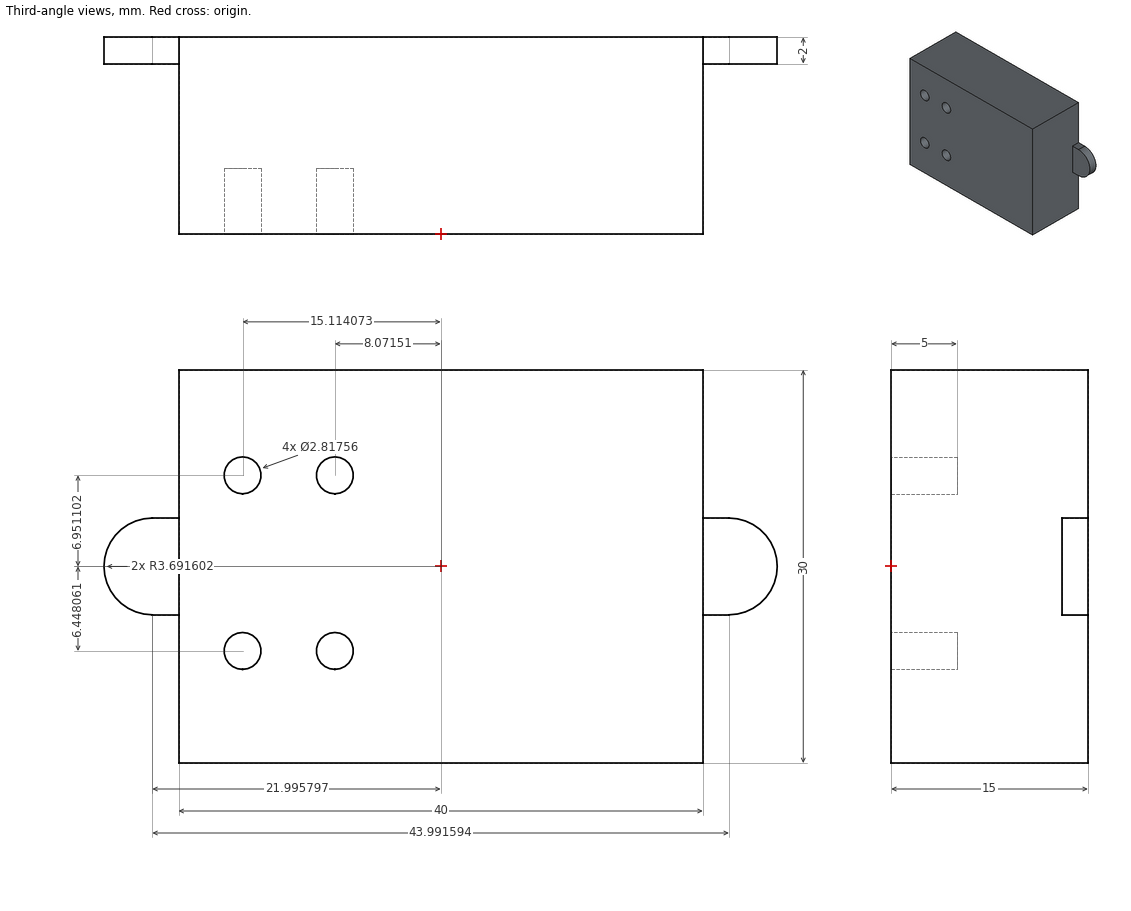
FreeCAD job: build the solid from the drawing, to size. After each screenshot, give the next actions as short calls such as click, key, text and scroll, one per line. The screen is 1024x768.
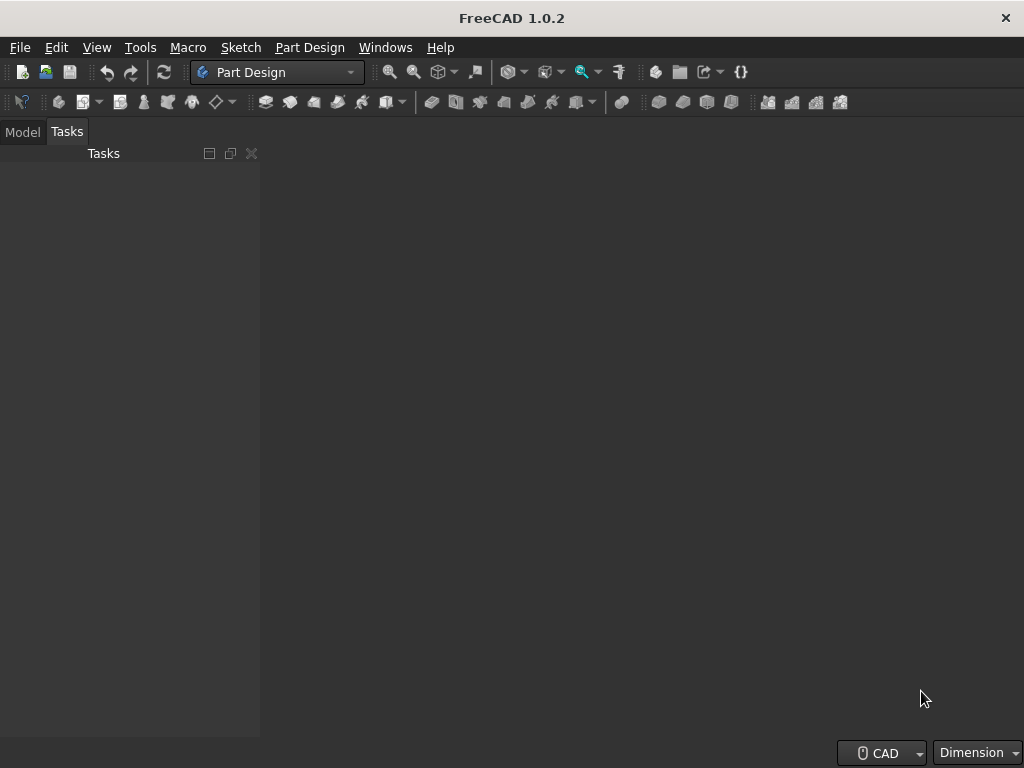
click(524, 72)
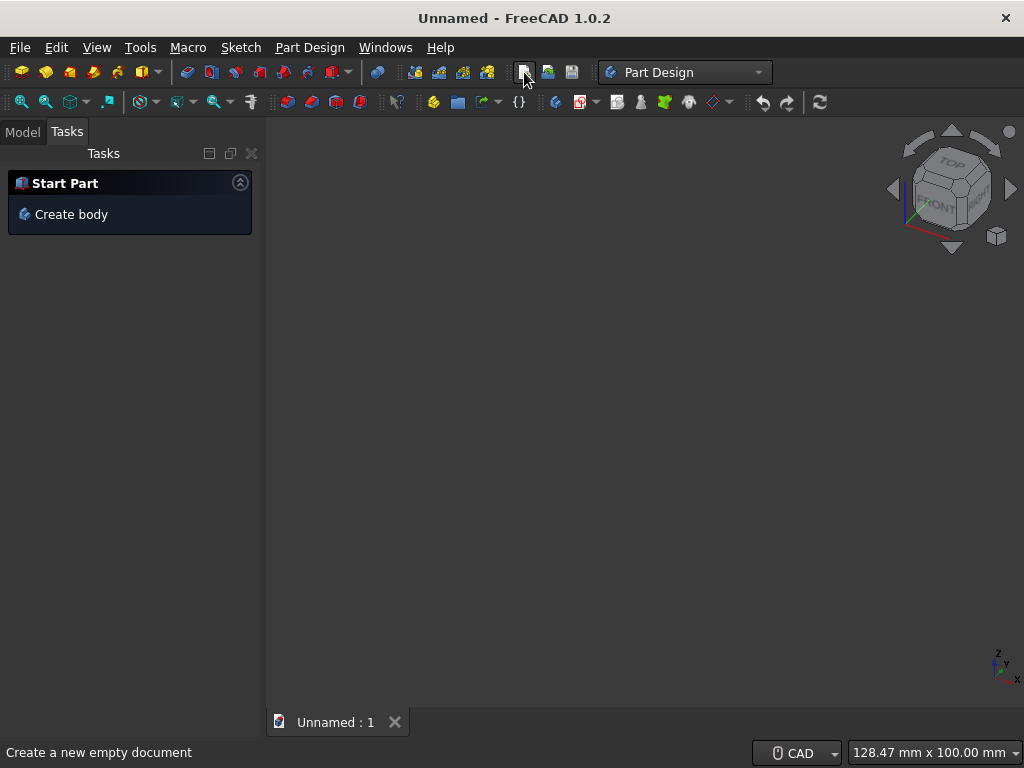
click(580, 102)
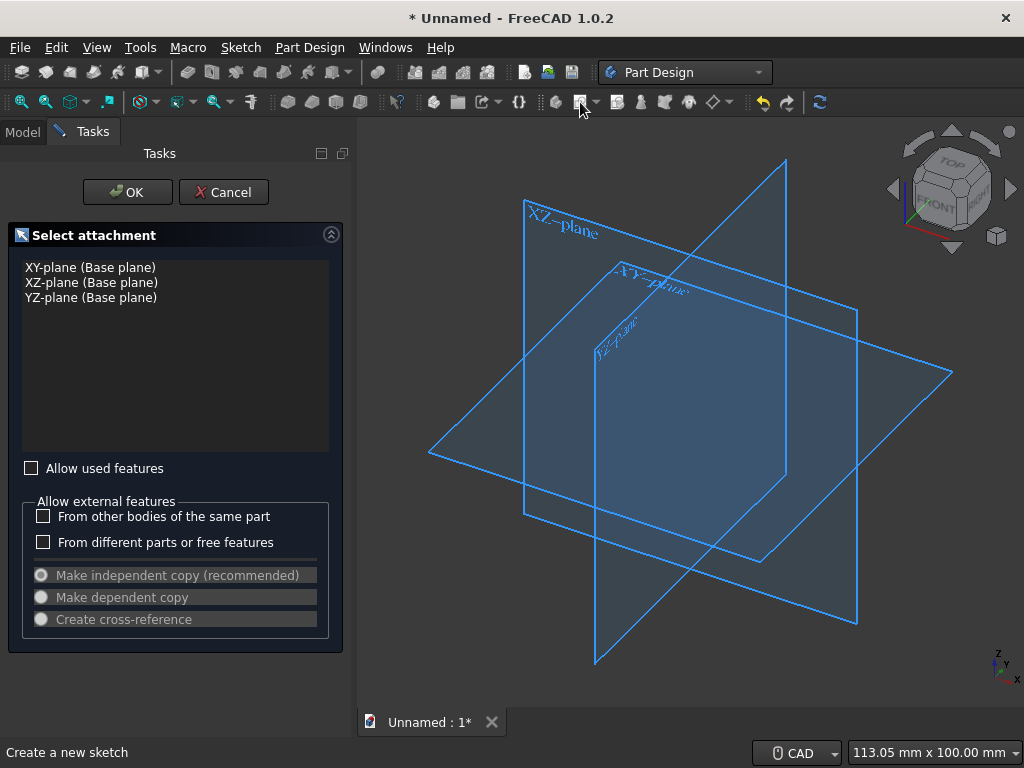
click(82, 282)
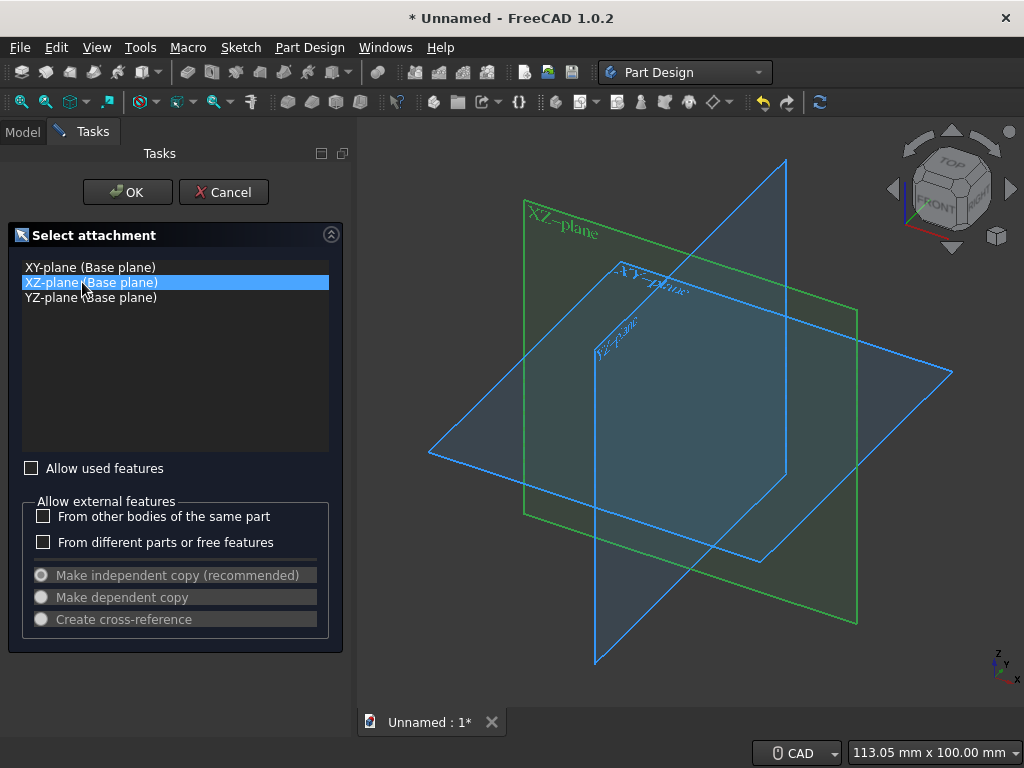
click(128, 192)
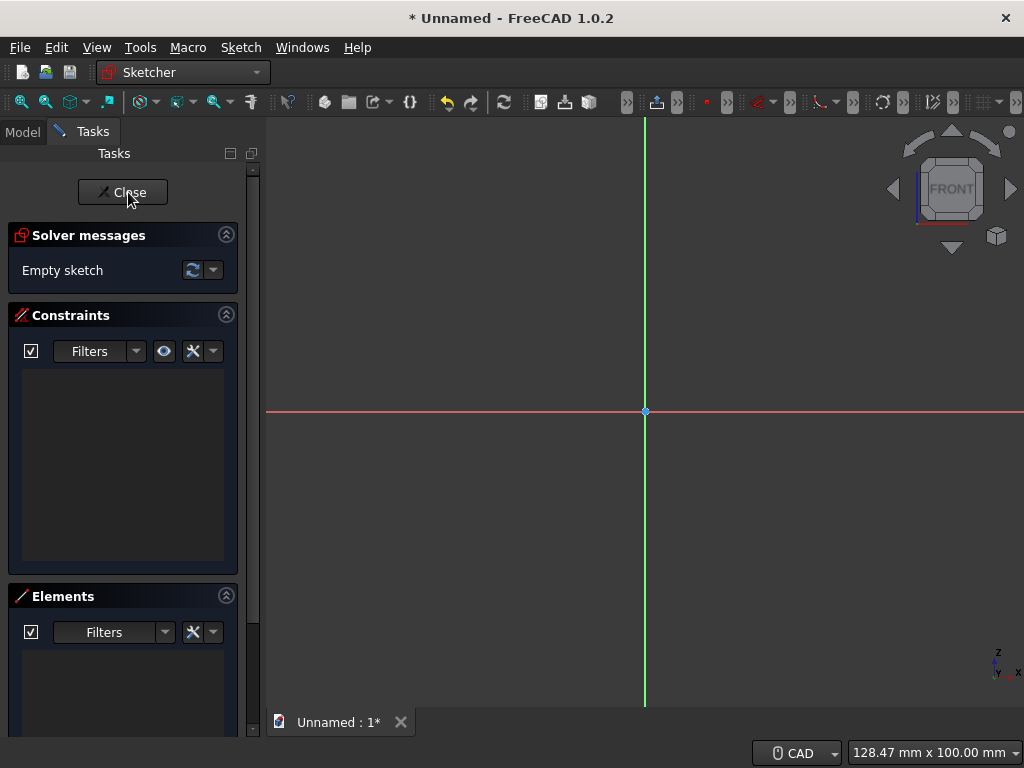
scroll(728, 412, up, 3)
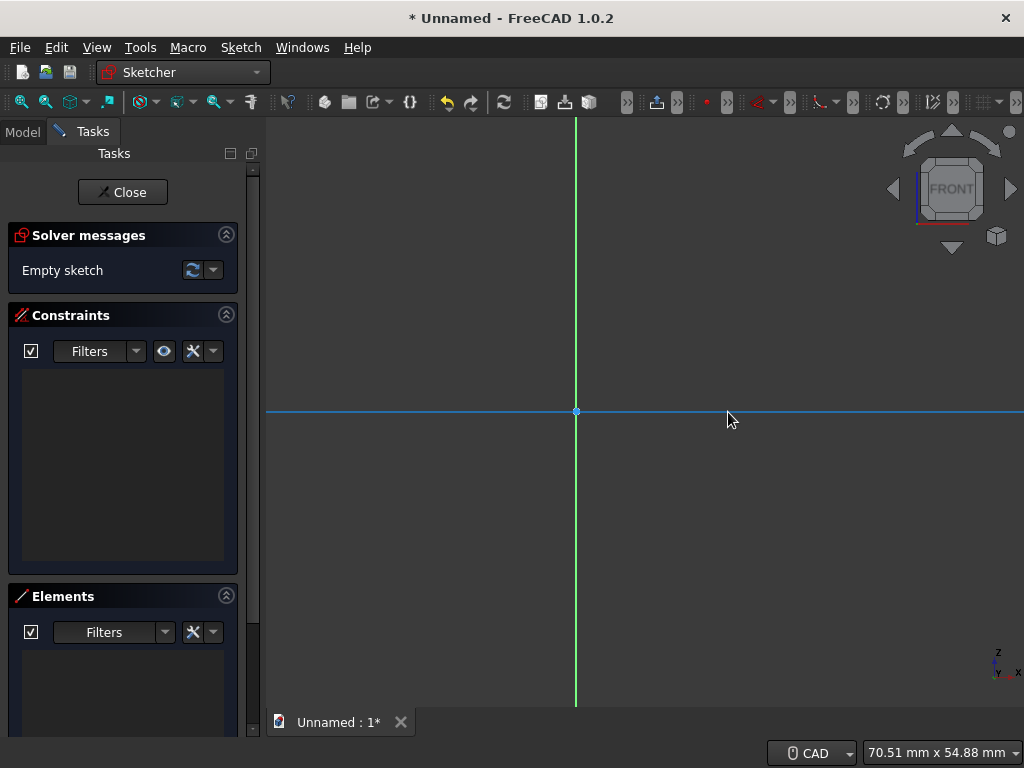
key(g)
key(v)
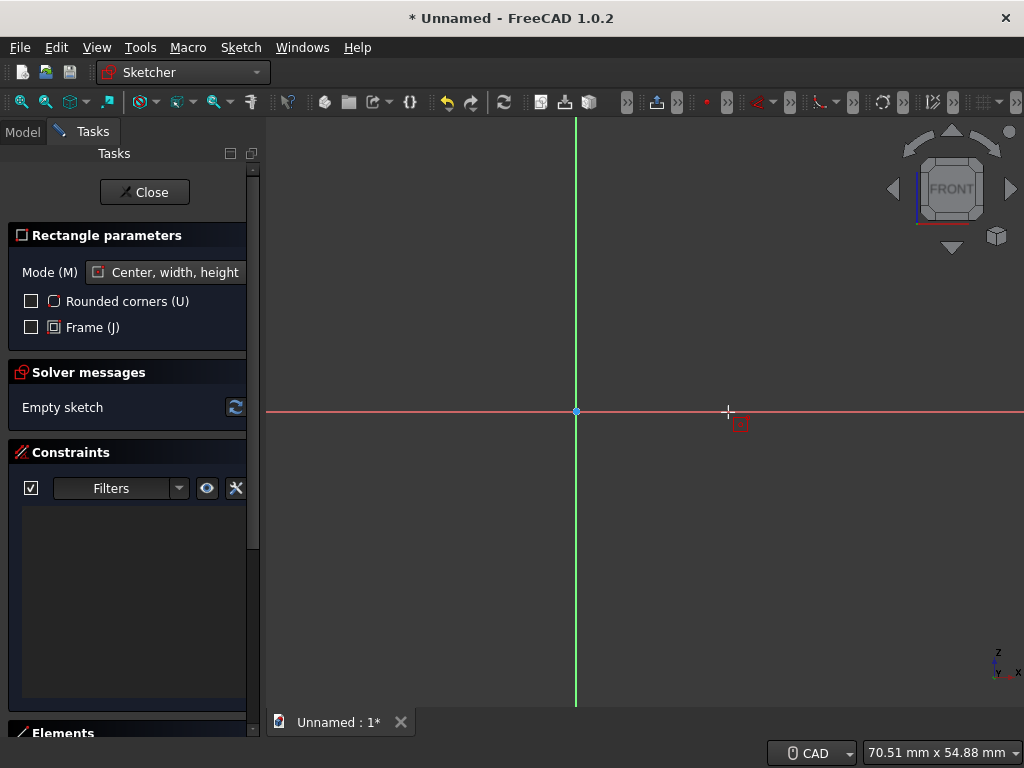
click(576, 412)
click(791, 250)
key(Escape)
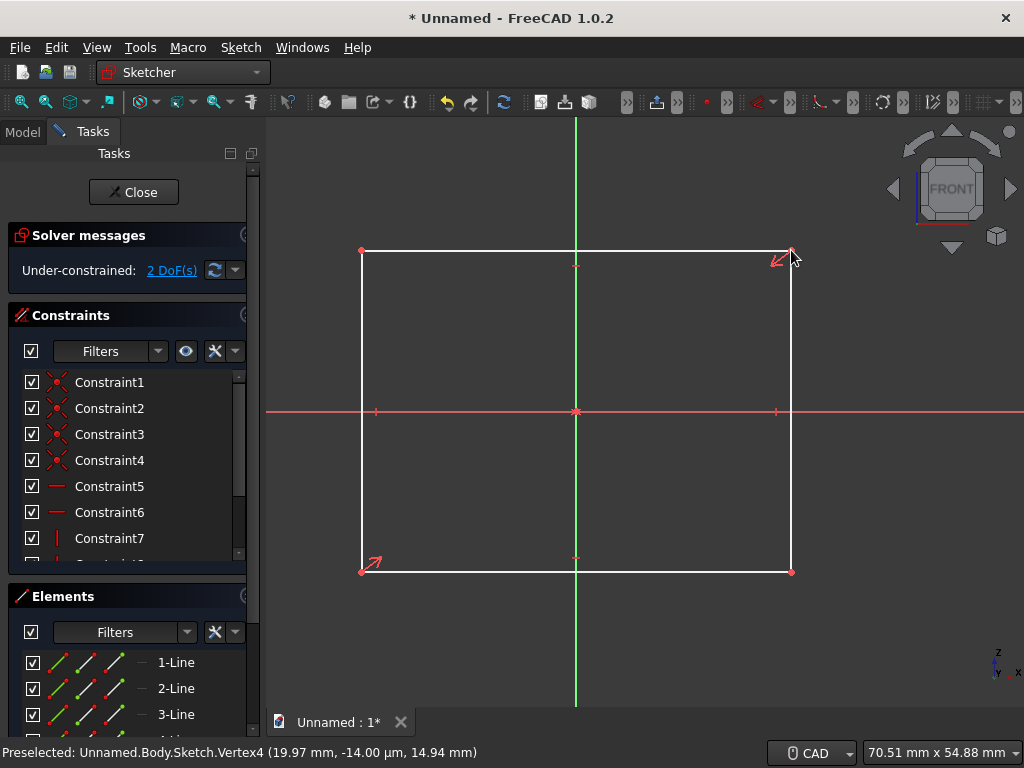
key(d)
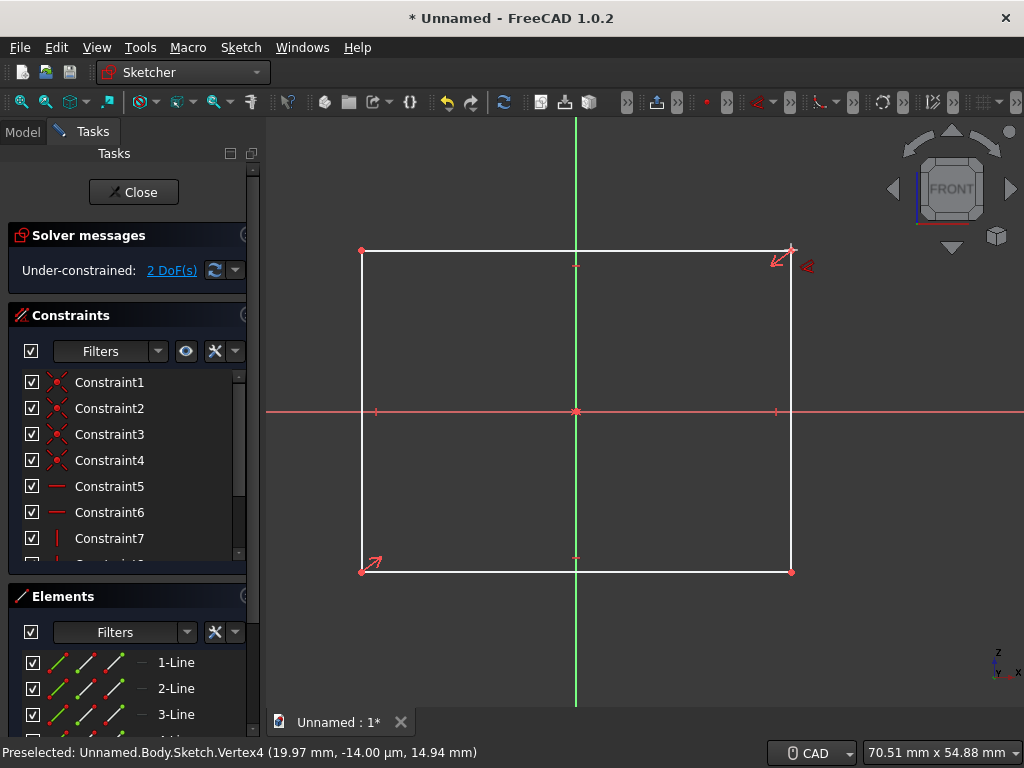
click(490, 572)
click(477, 606)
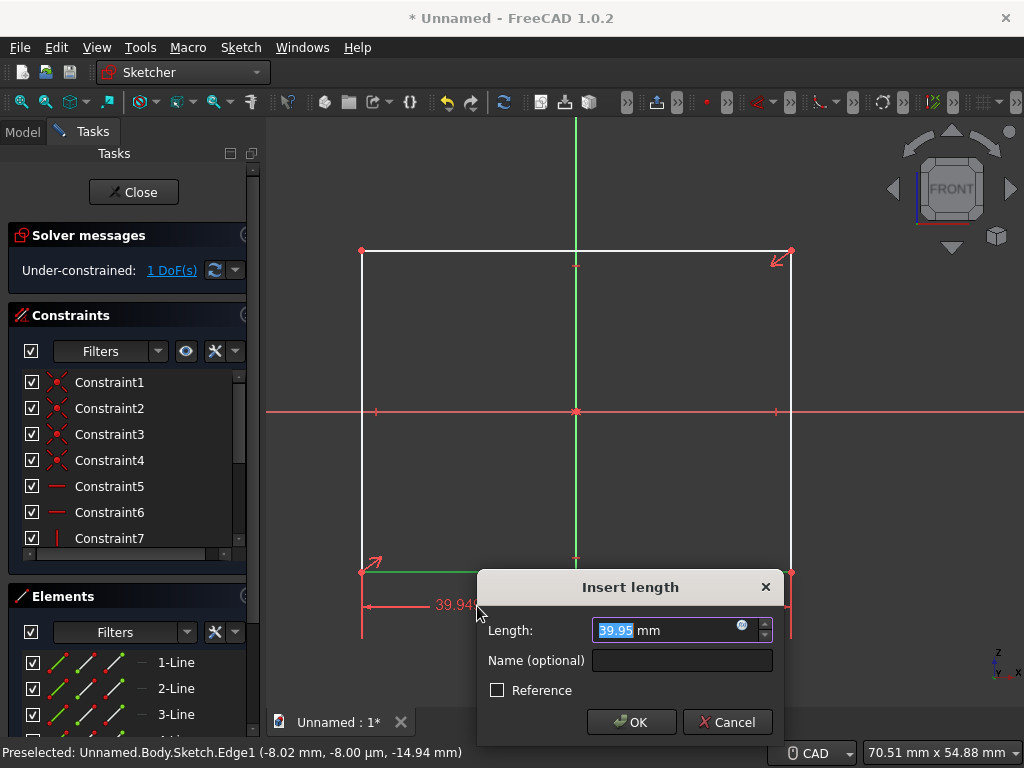
text(40)
key(Return)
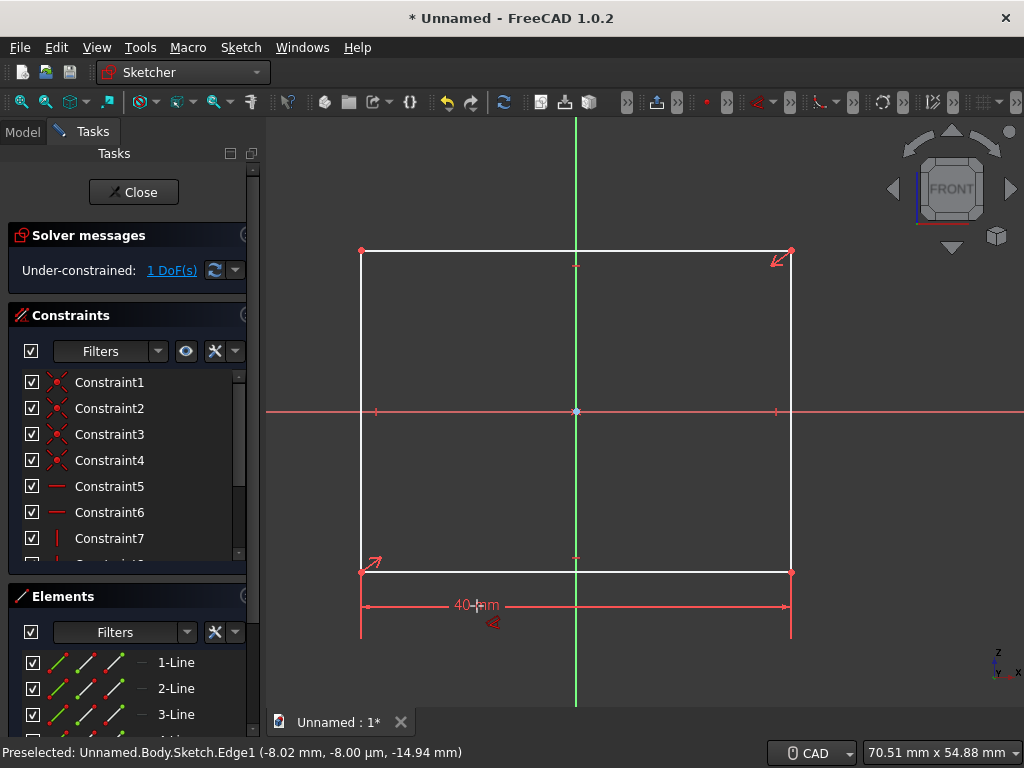
click(791, 476)
click(825, 338)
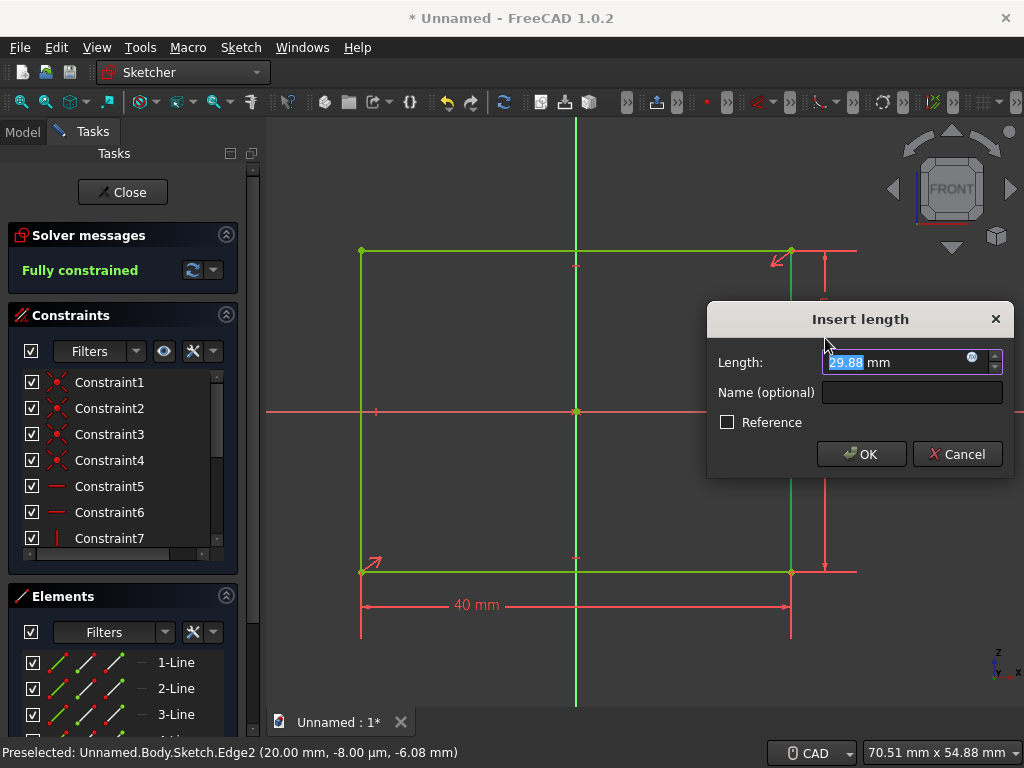
text(30)
key(Return)
key(Escape)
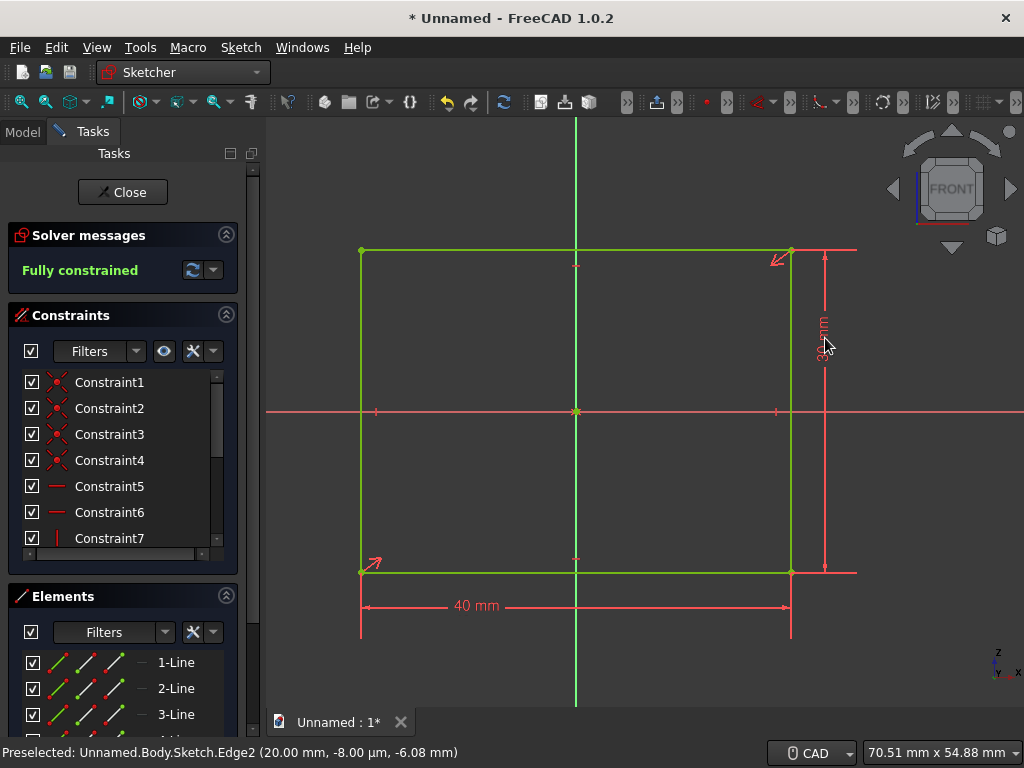
click(123, 192)